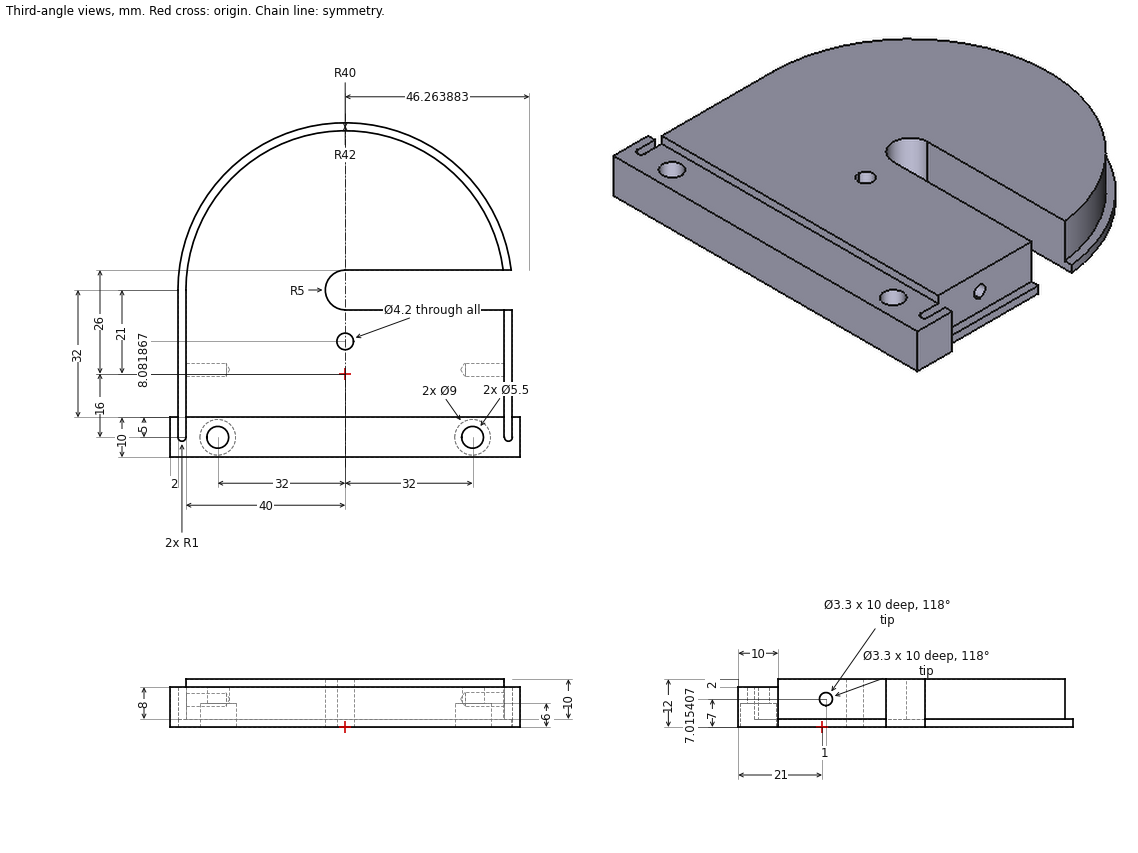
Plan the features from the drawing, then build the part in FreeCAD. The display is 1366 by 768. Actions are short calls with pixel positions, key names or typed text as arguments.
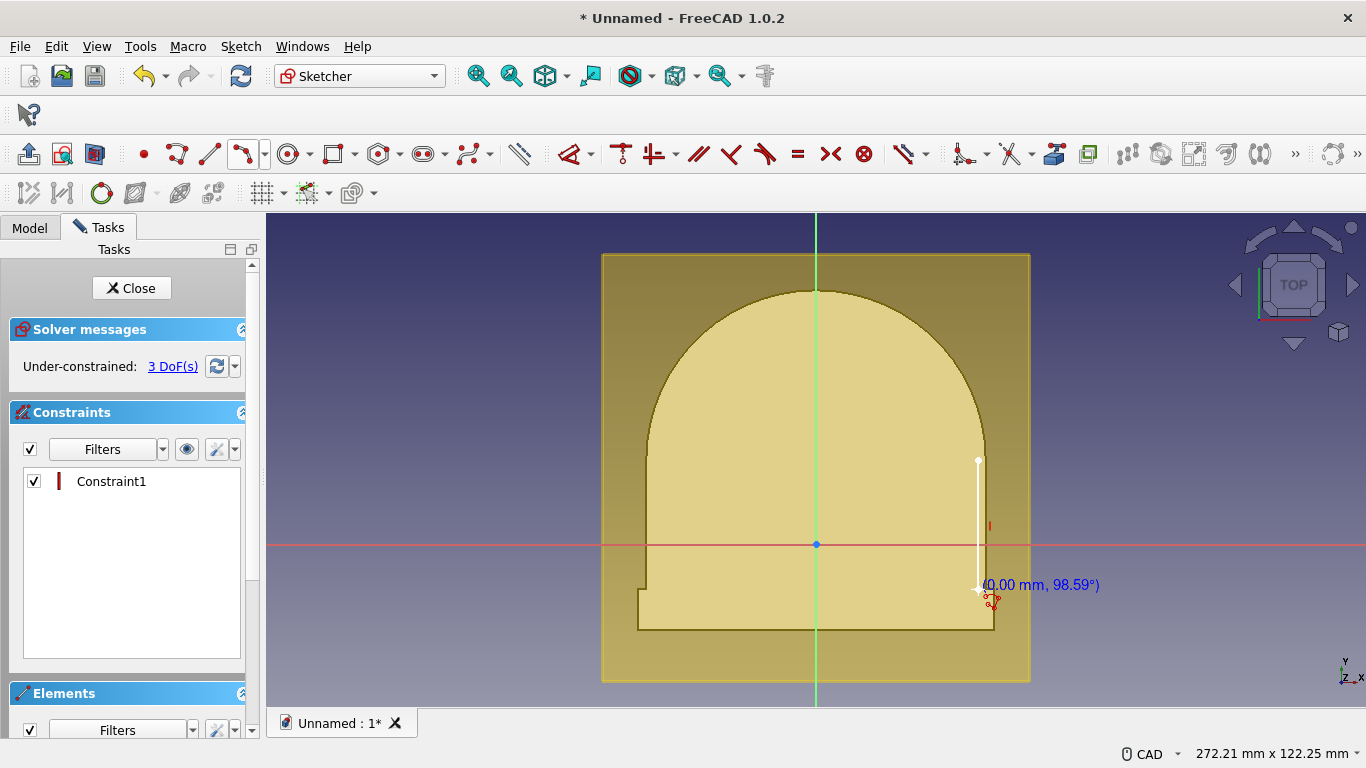
scroll(986, 589, up, 4)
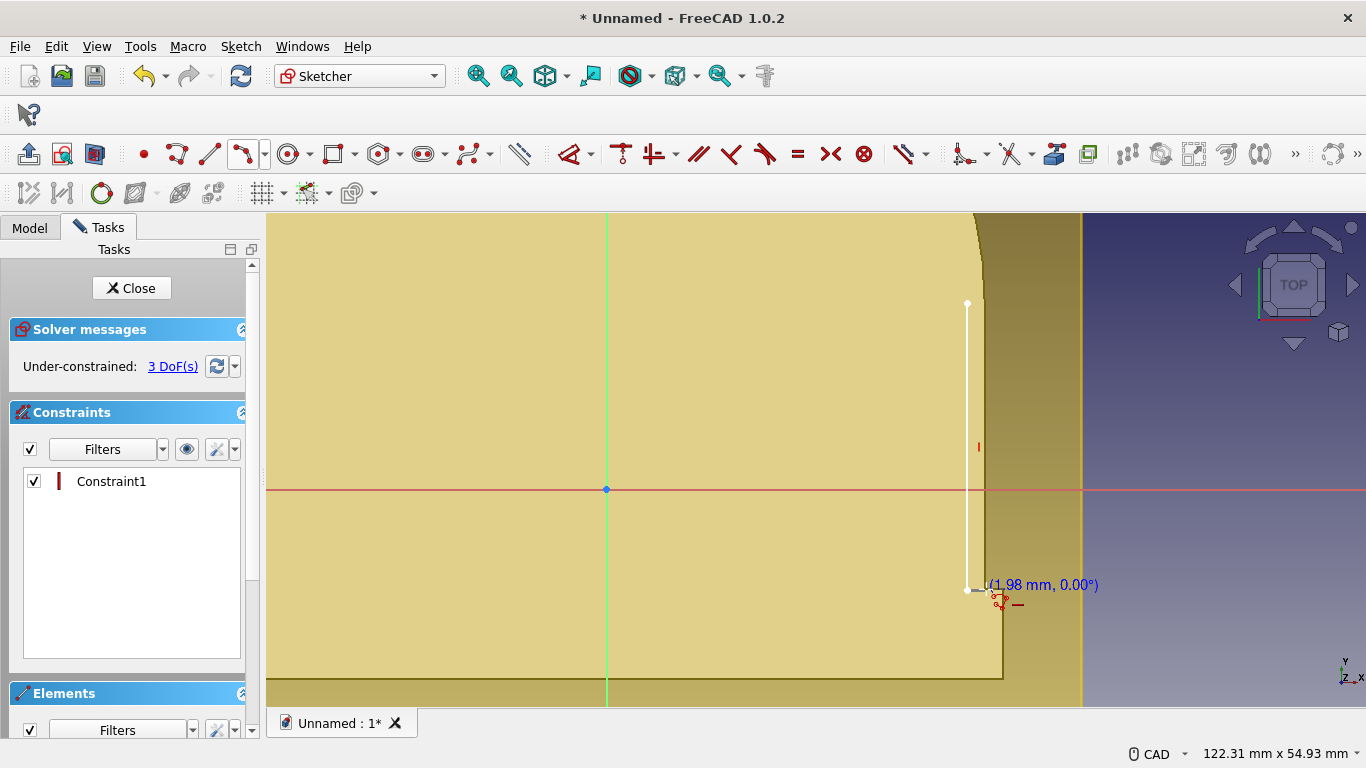
click(985, 588)
click(985, 301)
right_click(985, 301)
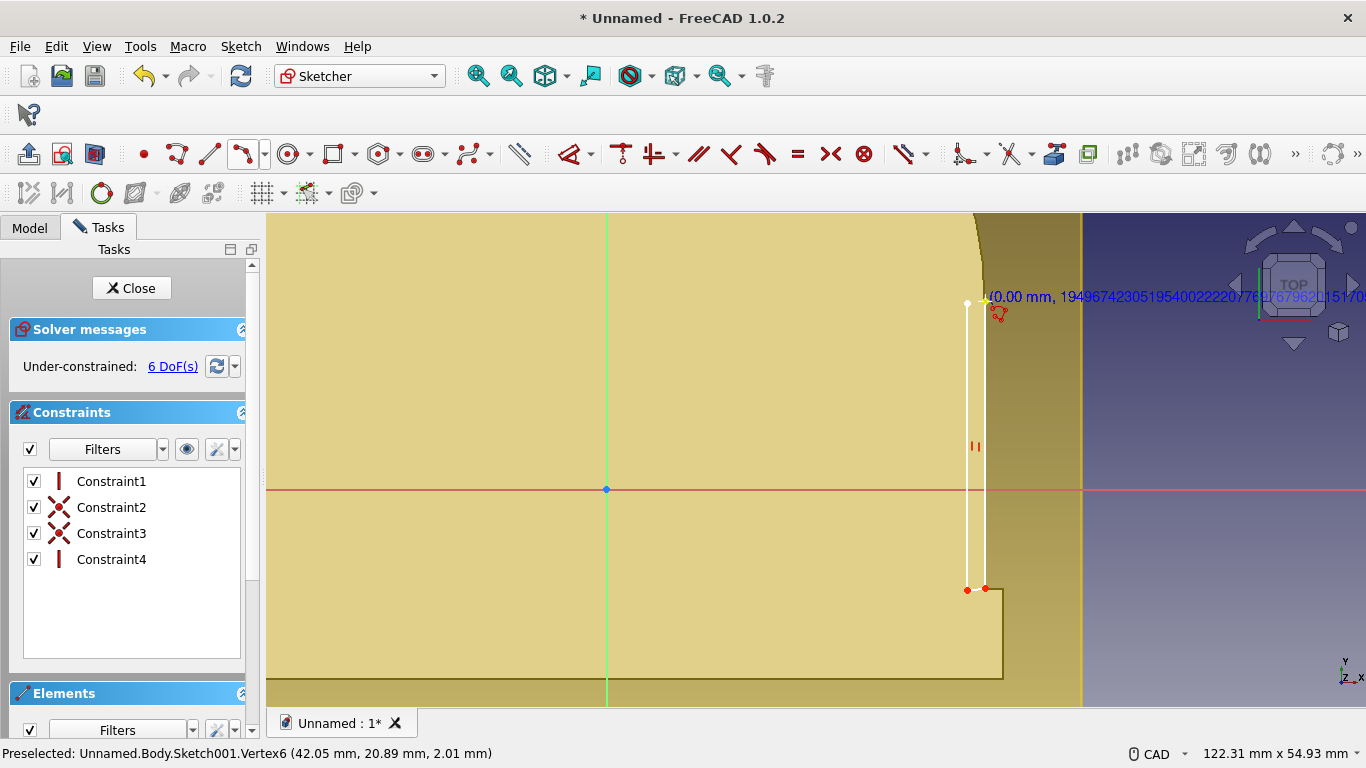
scroll(862, 626, down, 4)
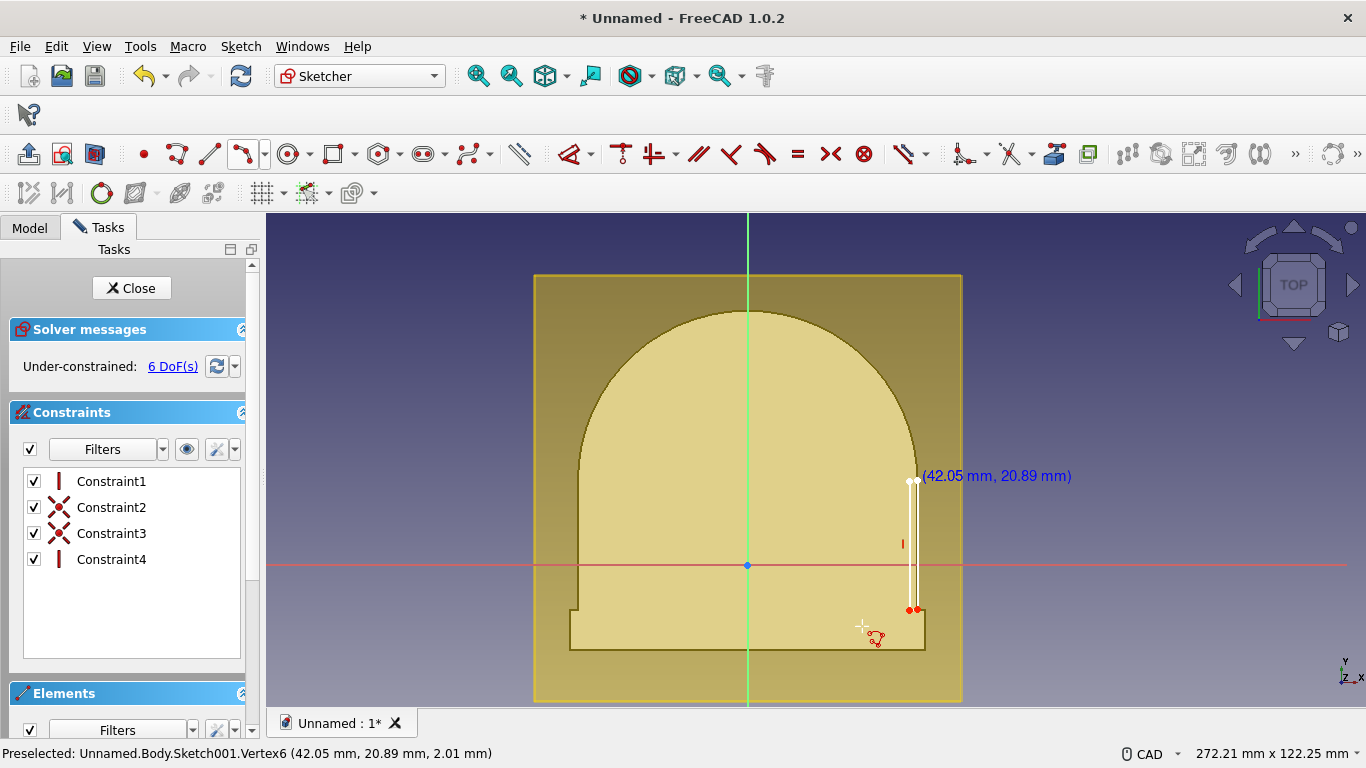
click(578, 480)
click(578, 610)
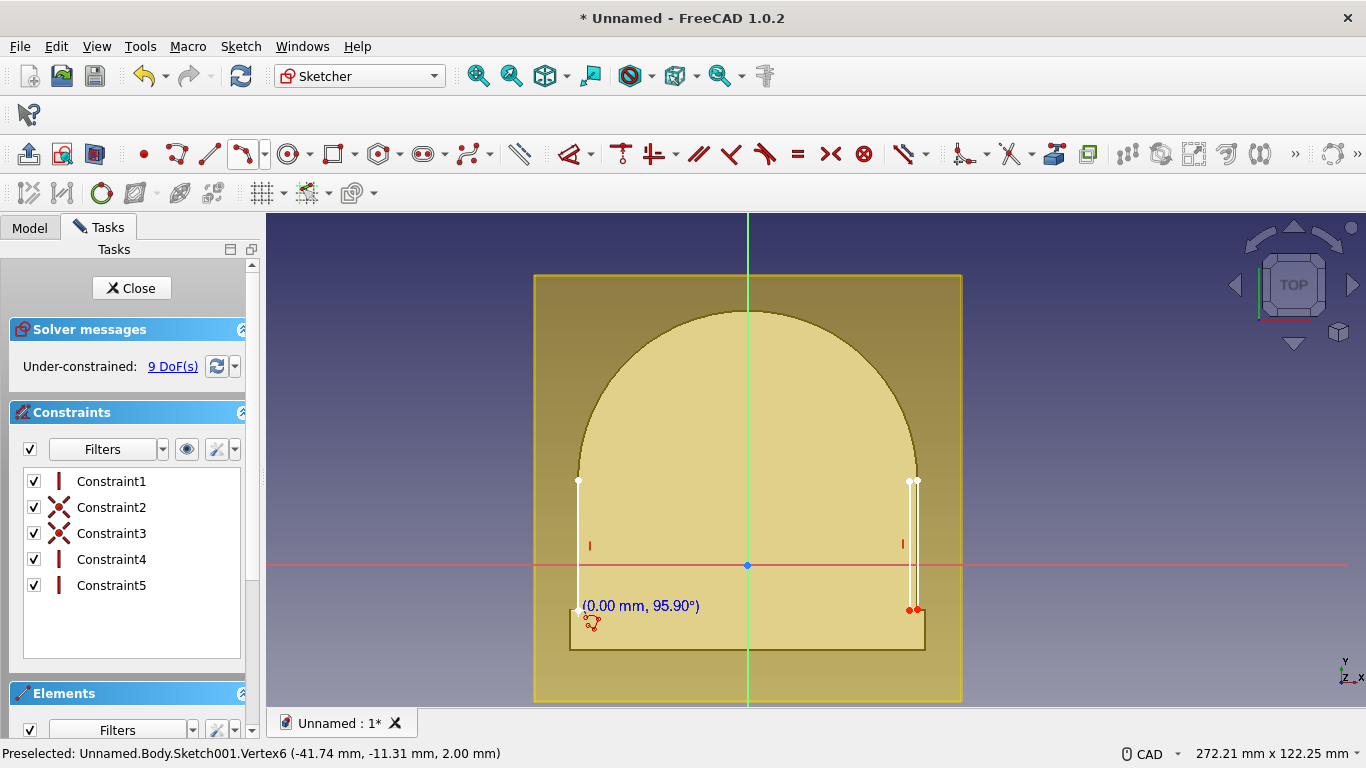
scroll(586, 610, up, 4)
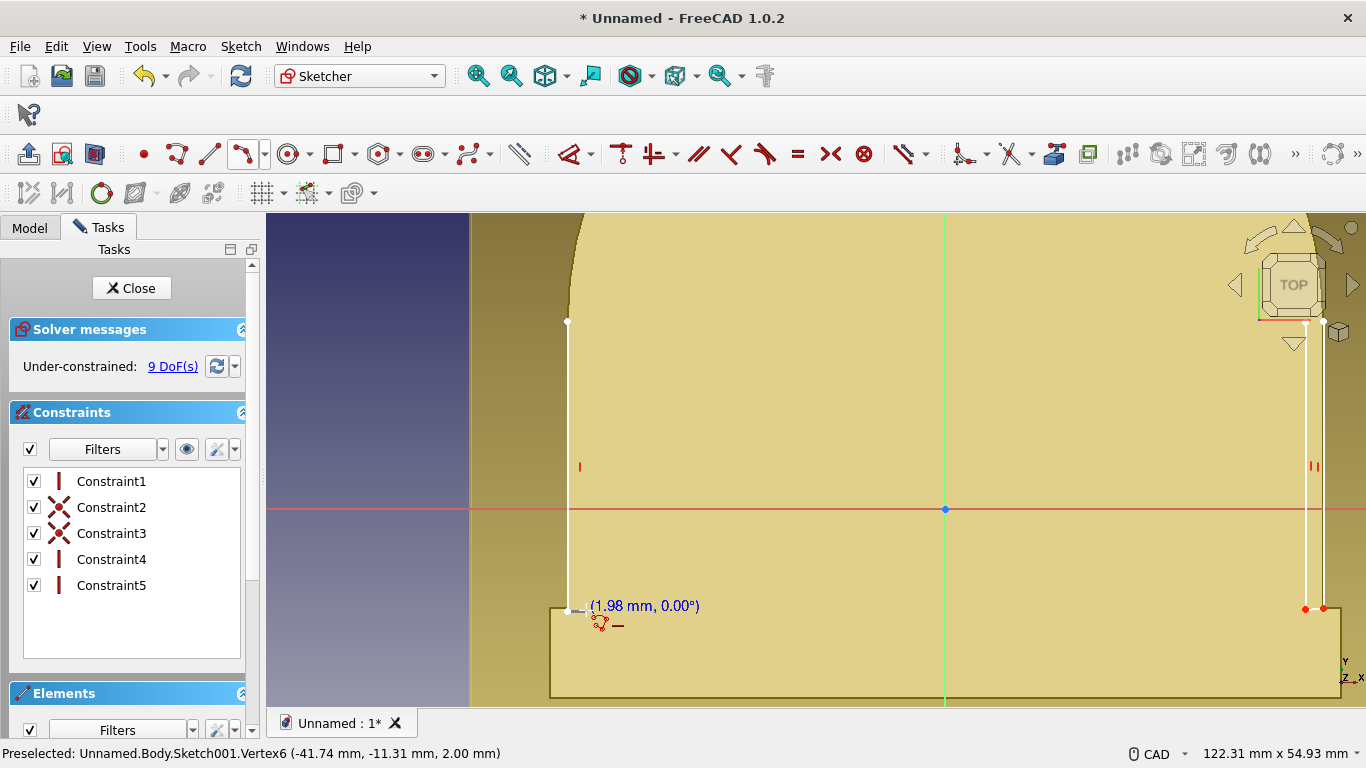
click(586, 609)
click(586, 321)
right_click(586, 321)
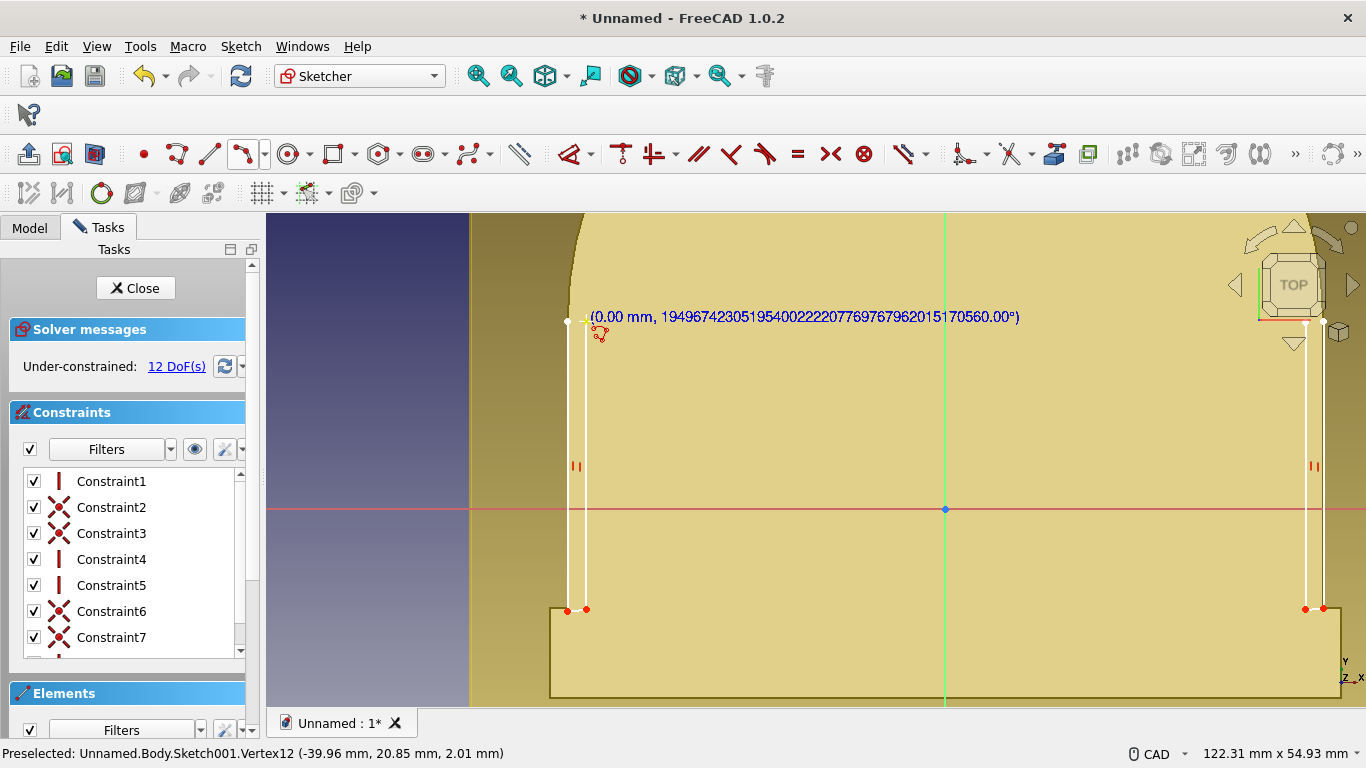
click(242, 154)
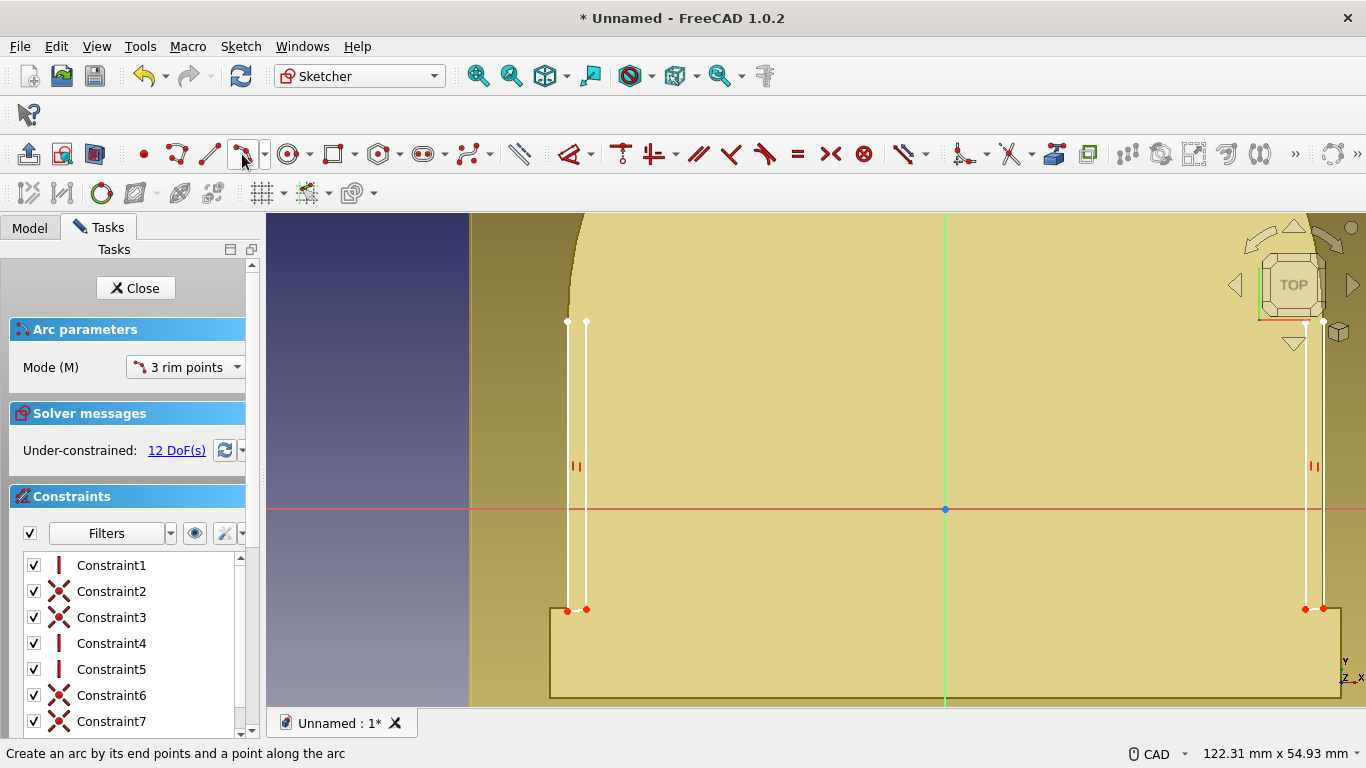
scroll(586, 610, down, 4)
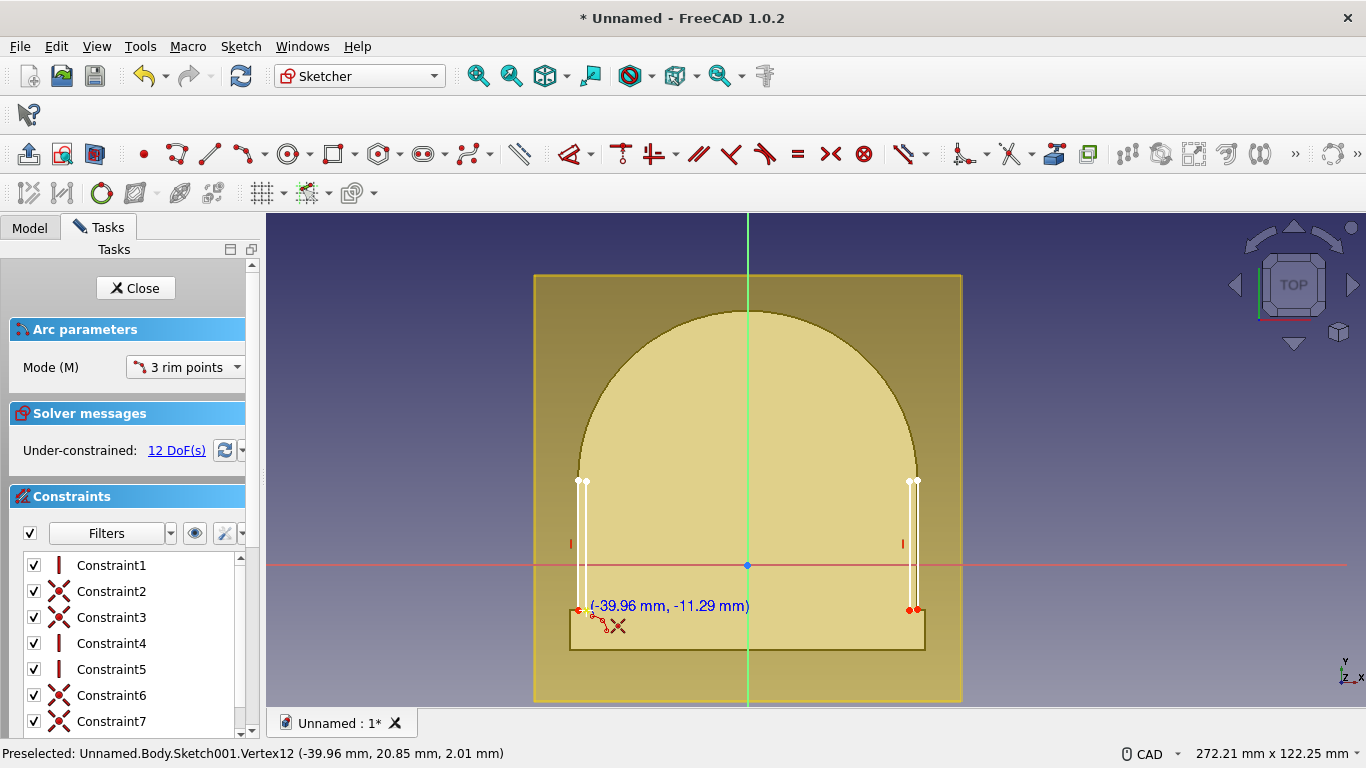
scroll(917, 480, up, 4)